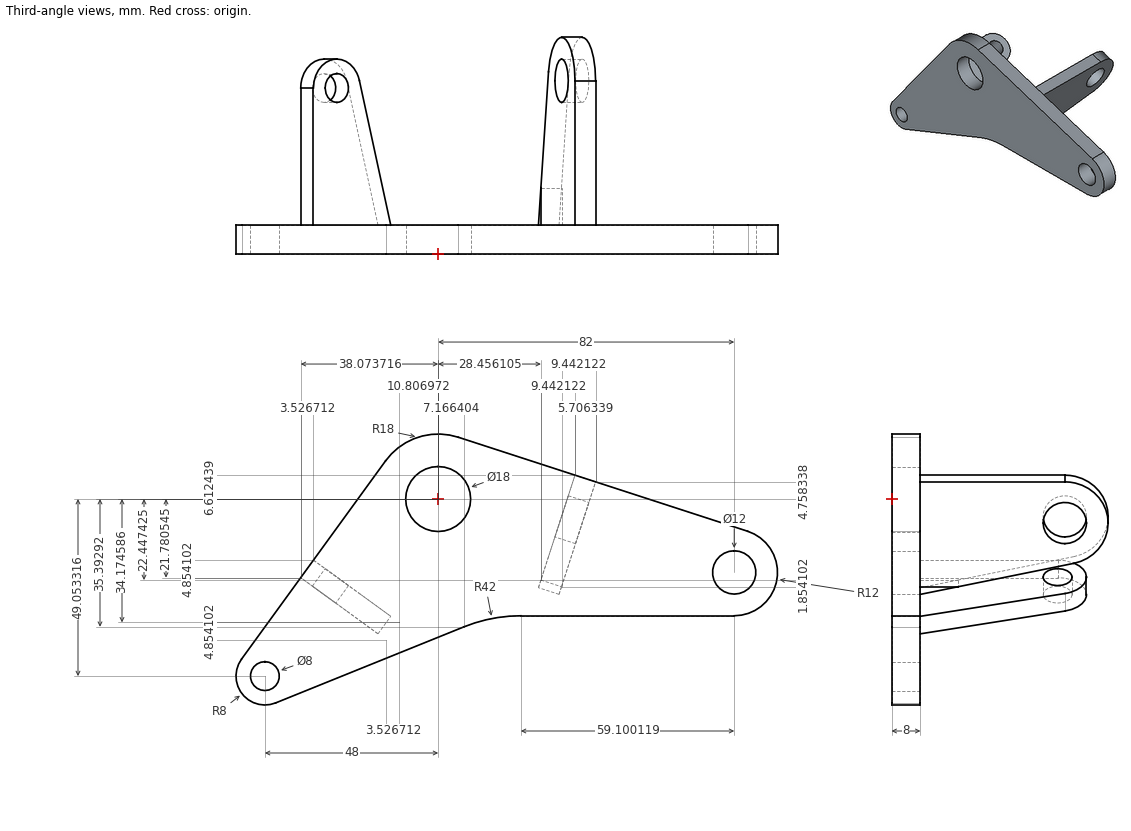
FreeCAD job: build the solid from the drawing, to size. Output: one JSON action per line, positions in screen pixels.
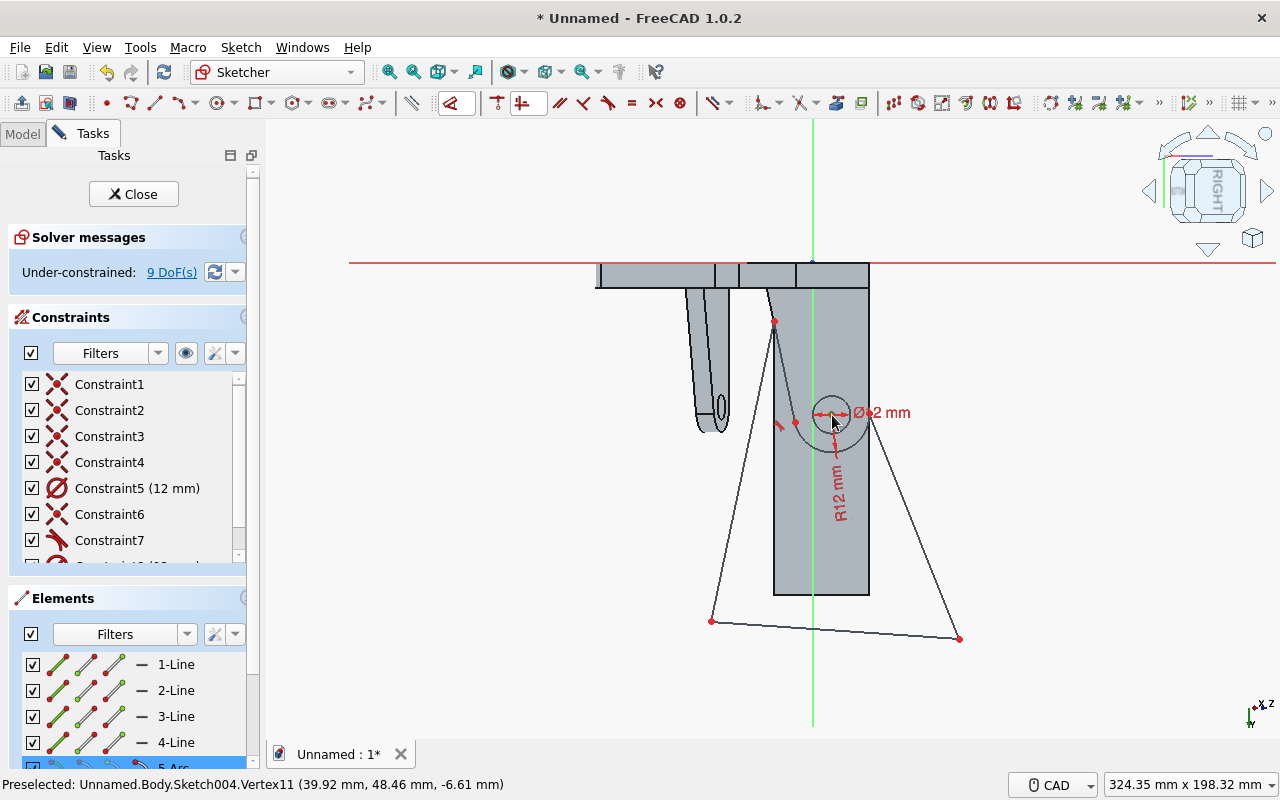
{"action": "key", "text": "i"}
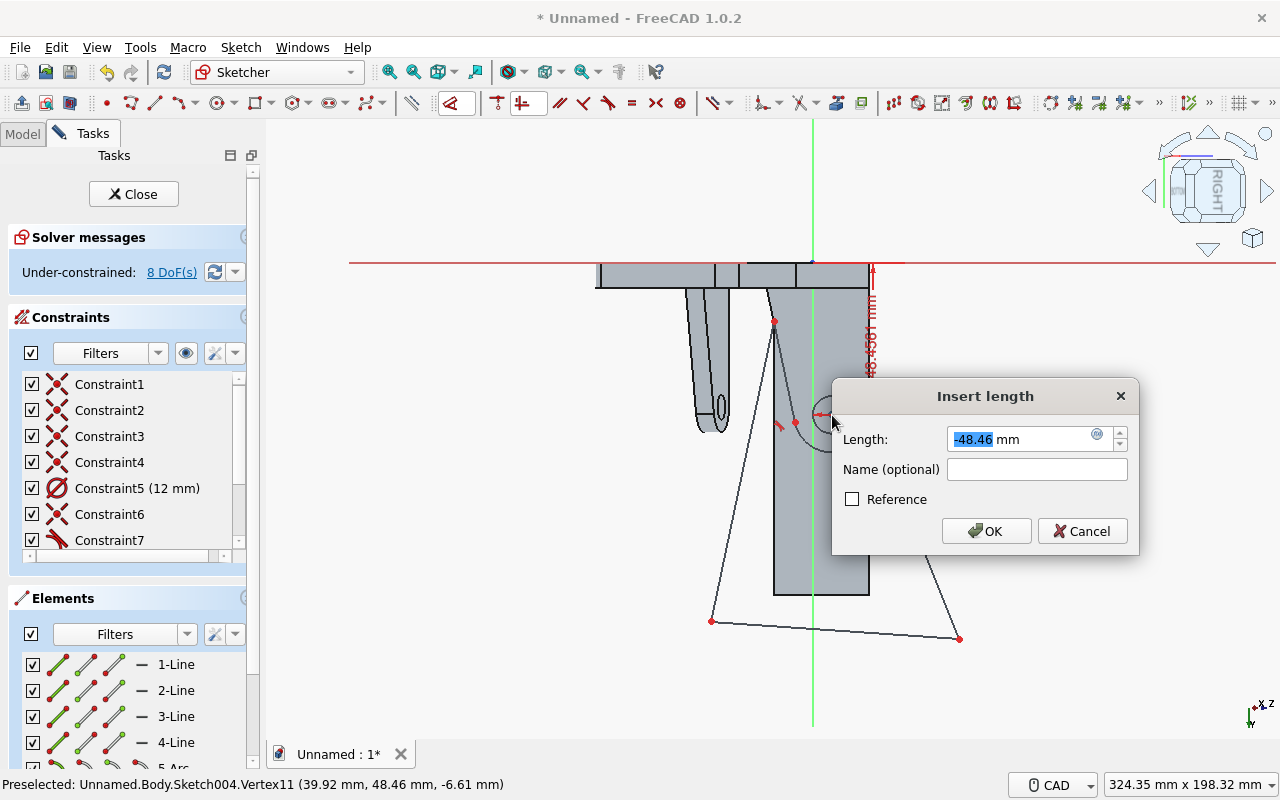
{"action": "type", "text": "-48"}
{"action": "key", "text": "Return"}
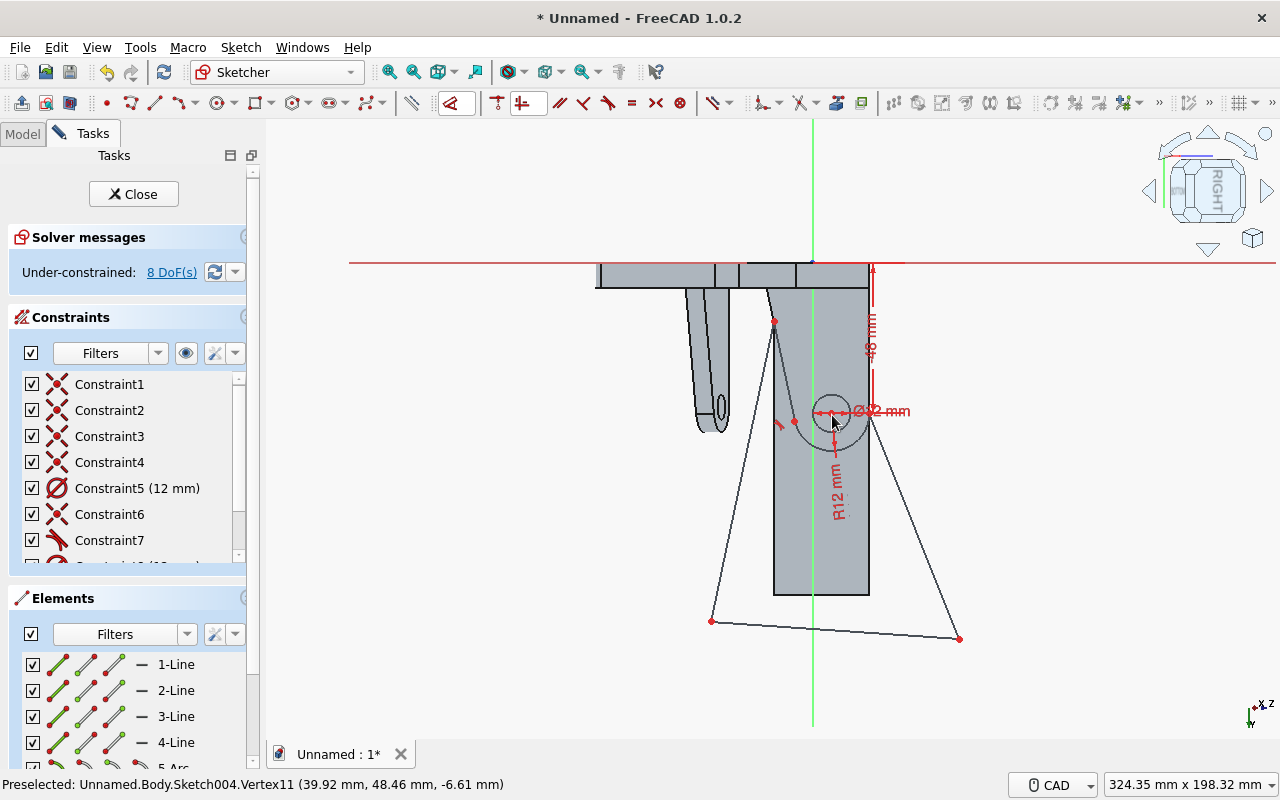
{"action": "left_click", "coordinate": [869, 414]}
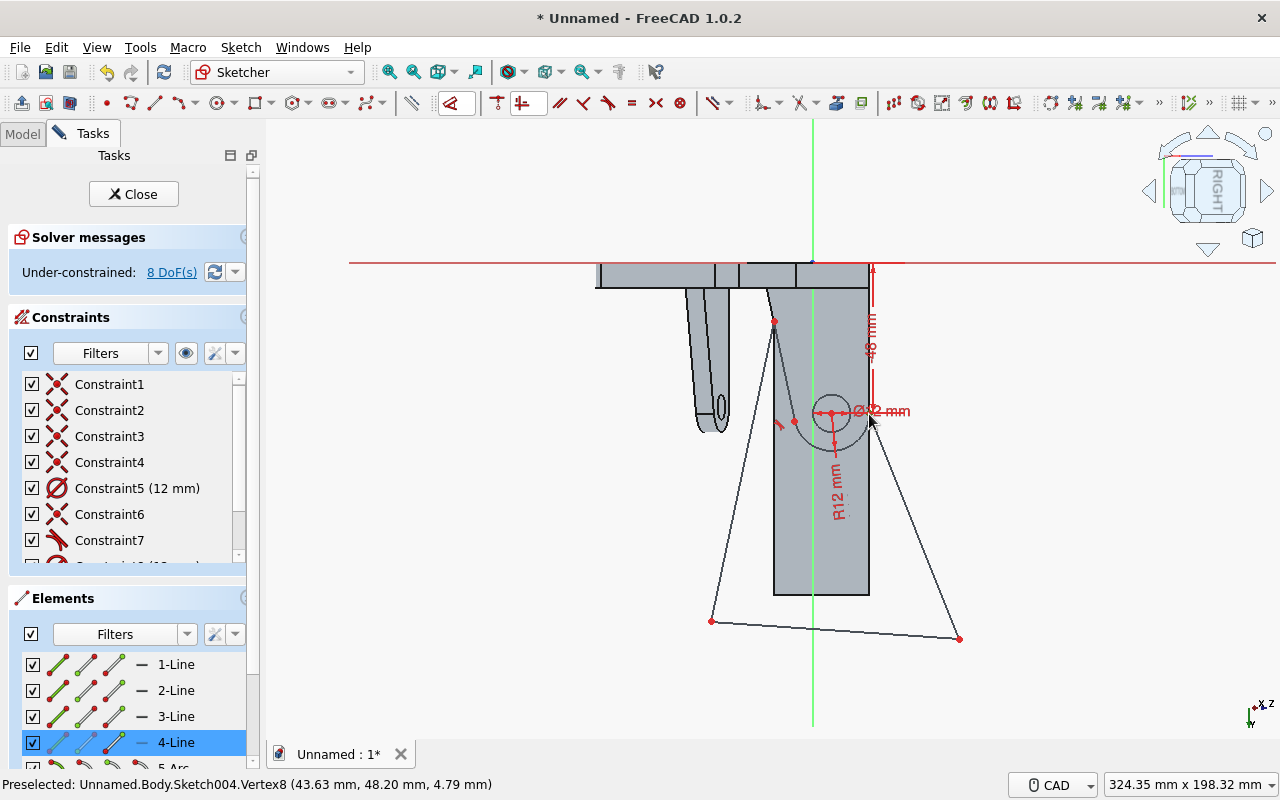
{"action": "key", "text": "i"}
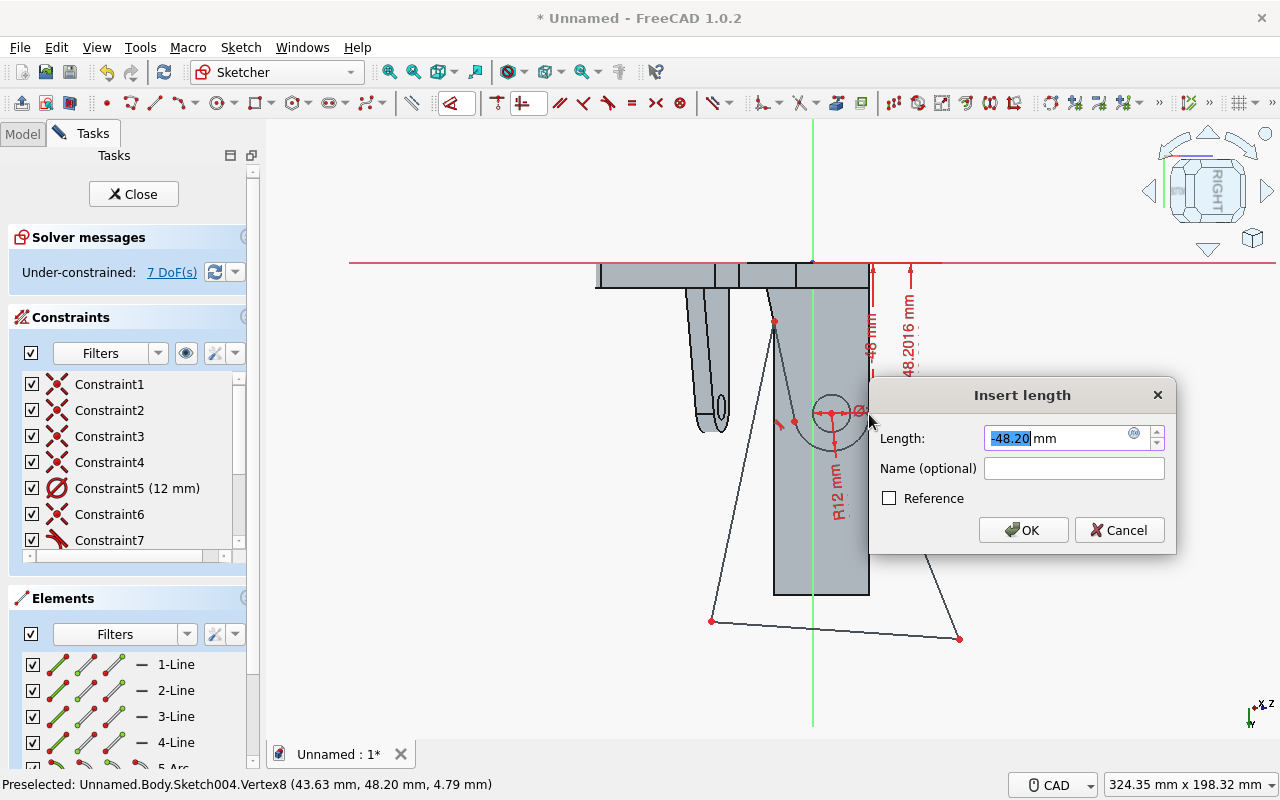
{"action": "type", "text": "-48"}
{"action": "key", "text": "Return"}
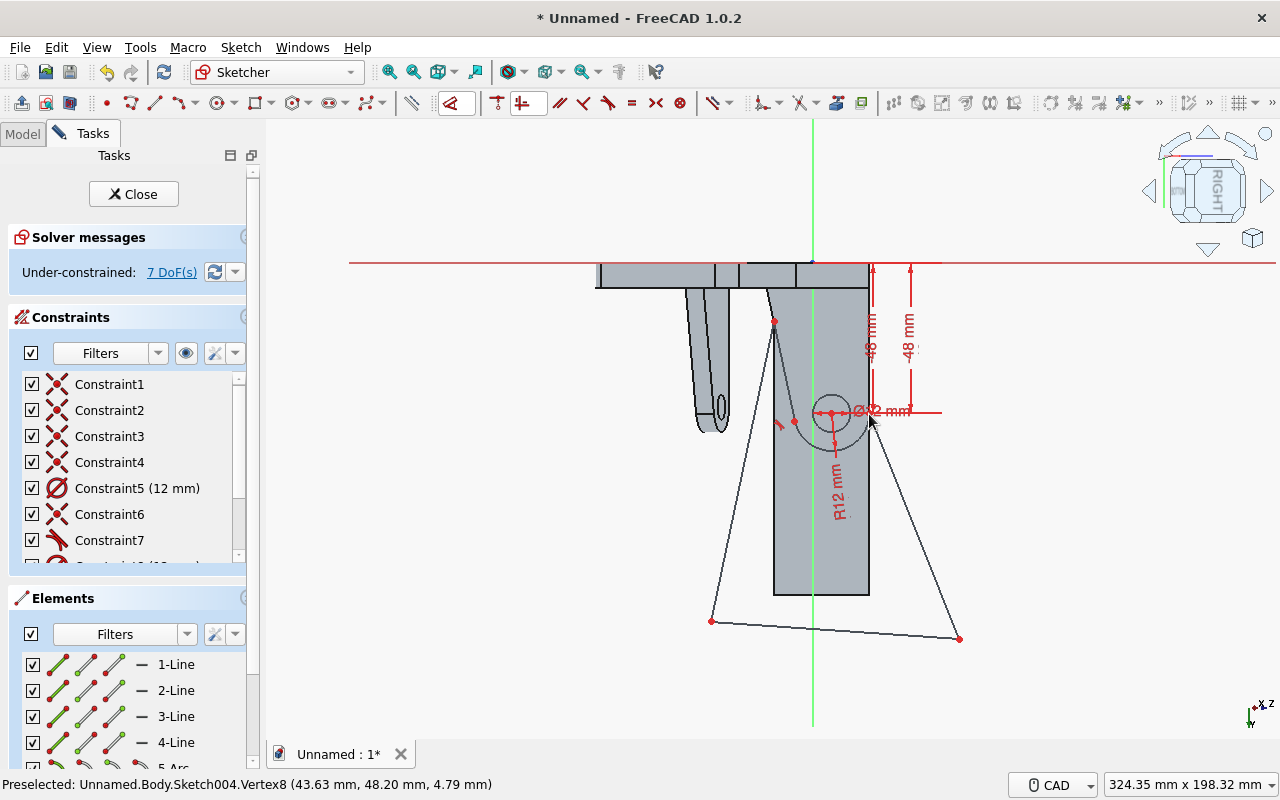
{"action": "scroll", "coordinate": [832, 413], "scroll_direction": "up", "scroll_amount": 4}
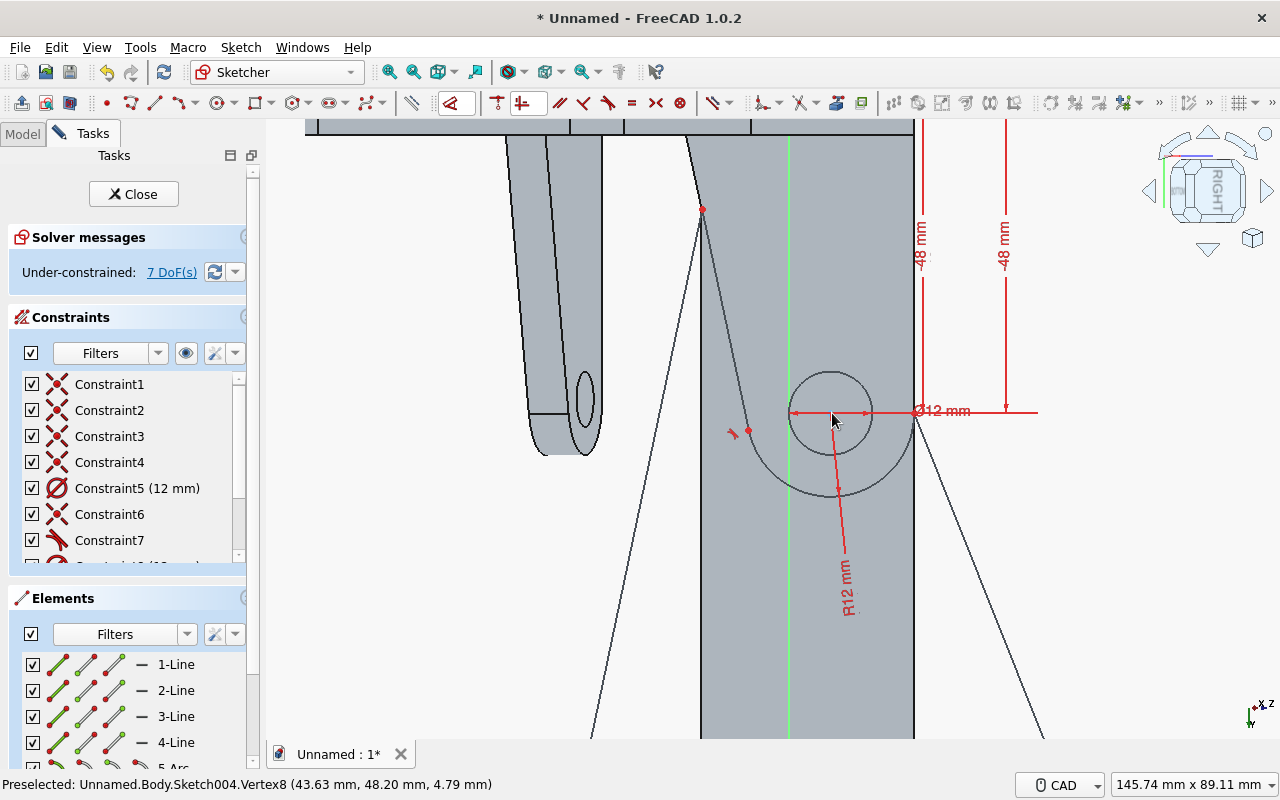
{"action": "left_click", "coordinate": [831, 413]}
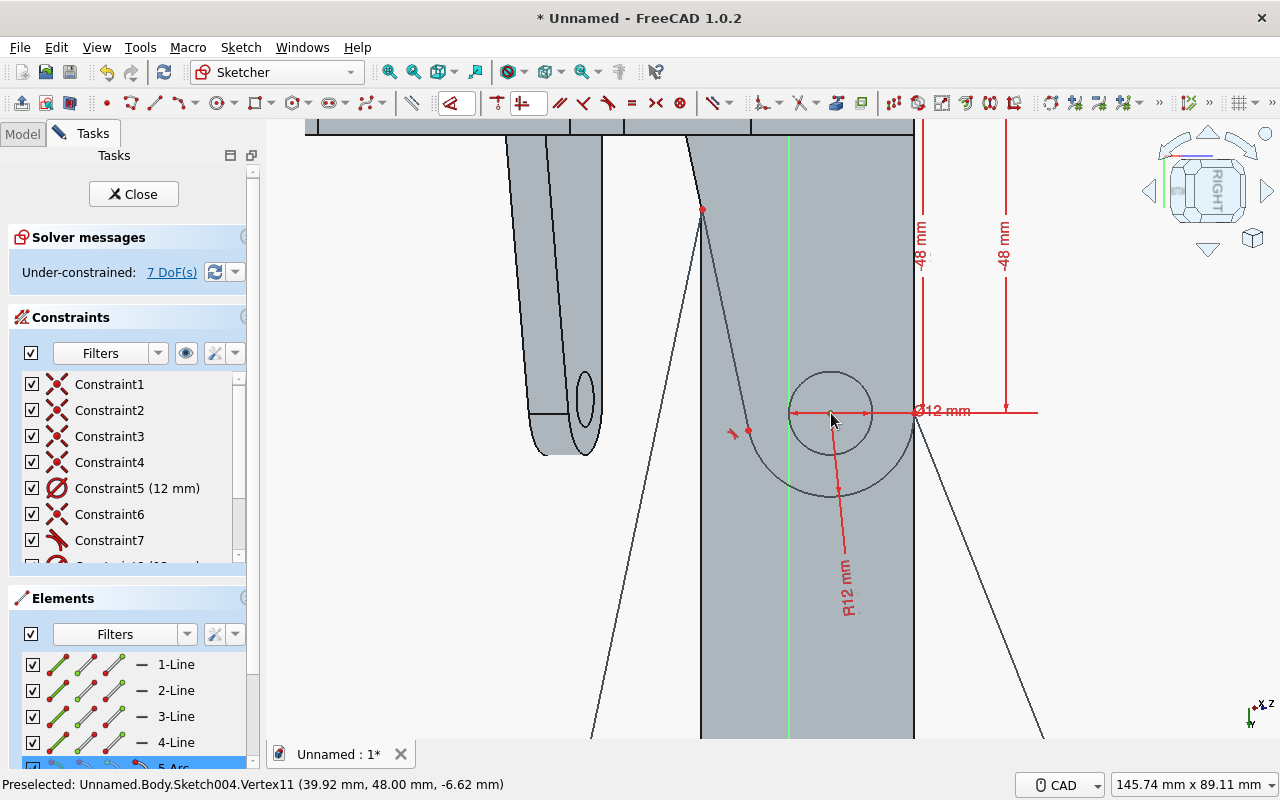
{"action": "left_click", "coordinate": [470, 104]}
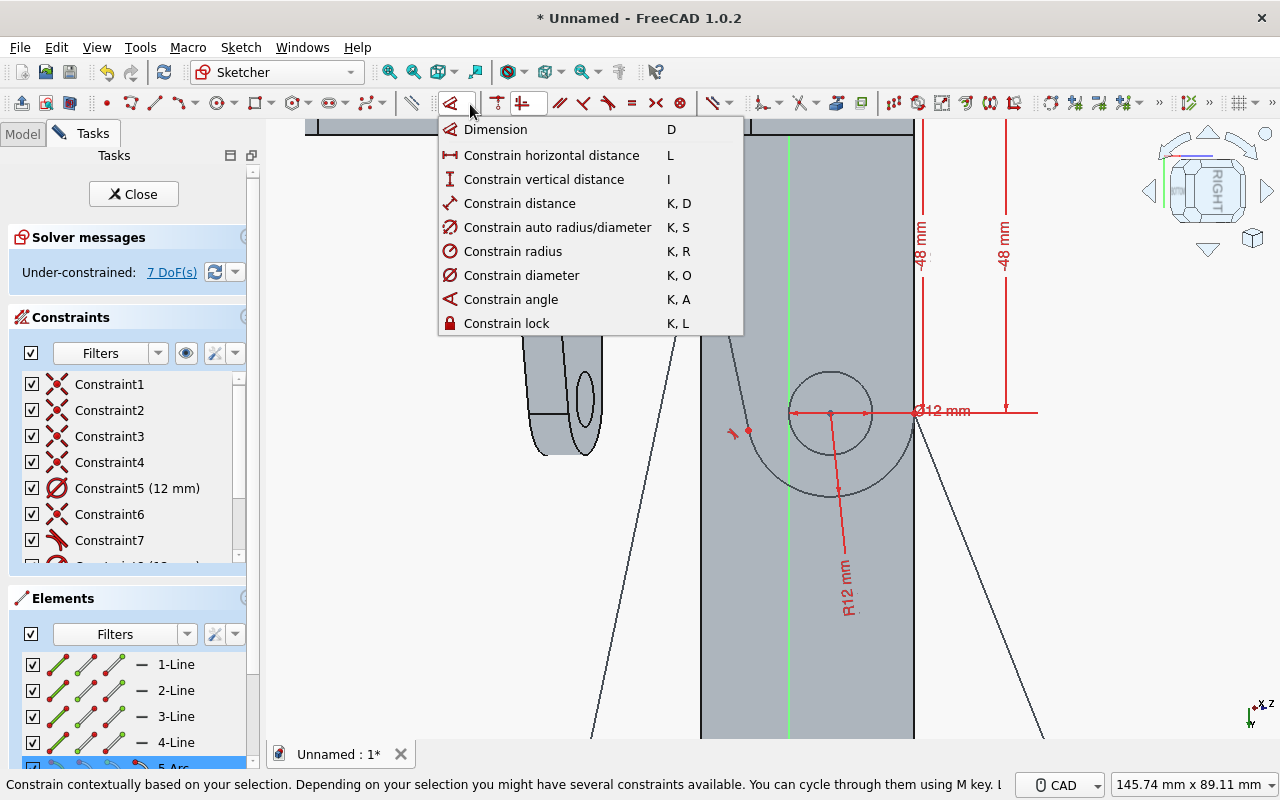
{"action": "left_click", "coordinate": [591, 155]}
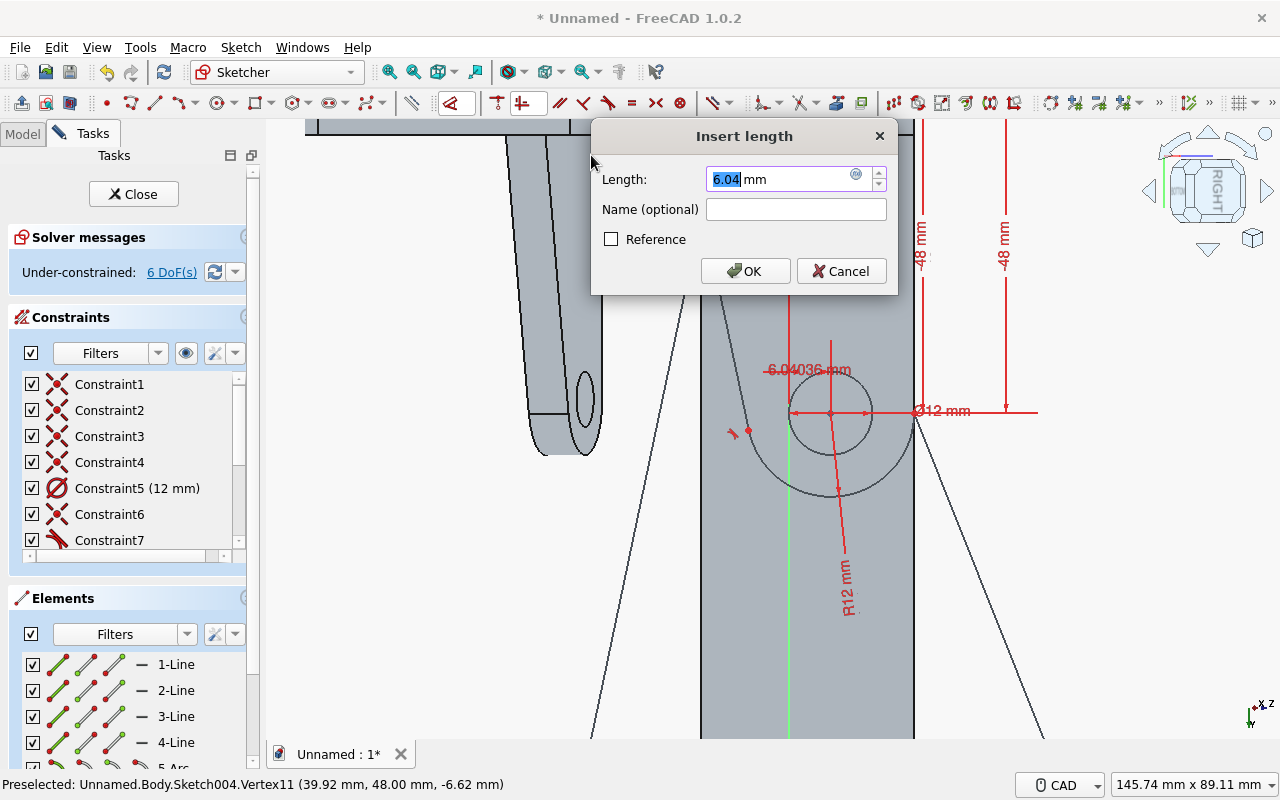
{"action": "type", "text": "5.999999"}
{"action": "key", "text": "Return"}